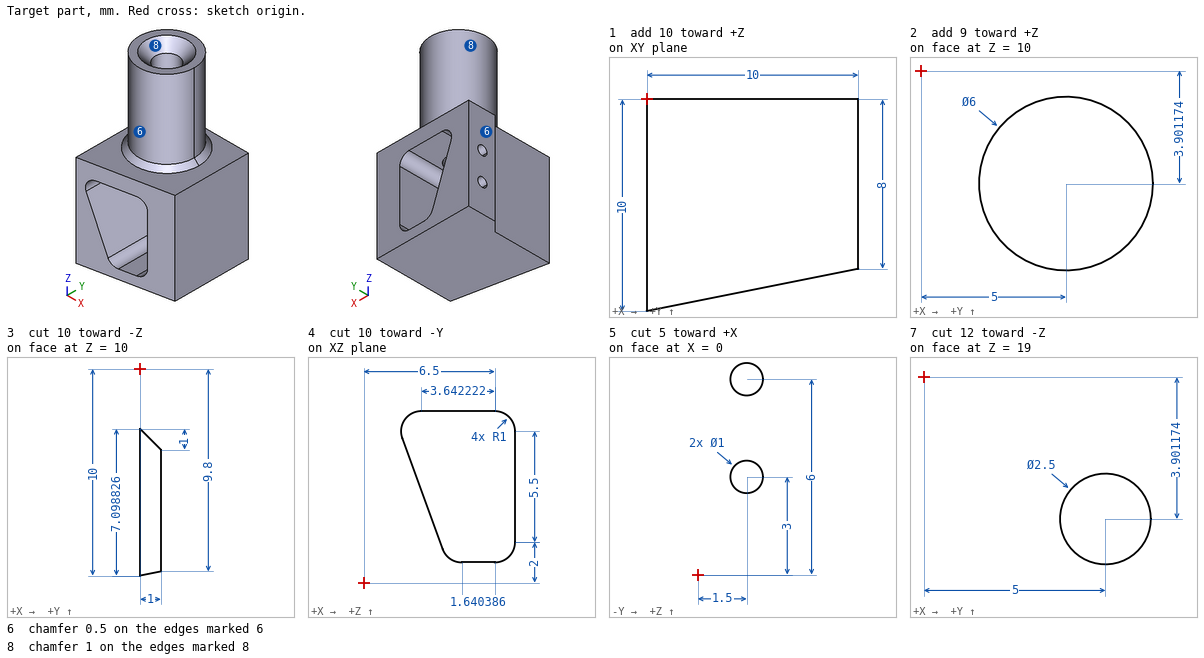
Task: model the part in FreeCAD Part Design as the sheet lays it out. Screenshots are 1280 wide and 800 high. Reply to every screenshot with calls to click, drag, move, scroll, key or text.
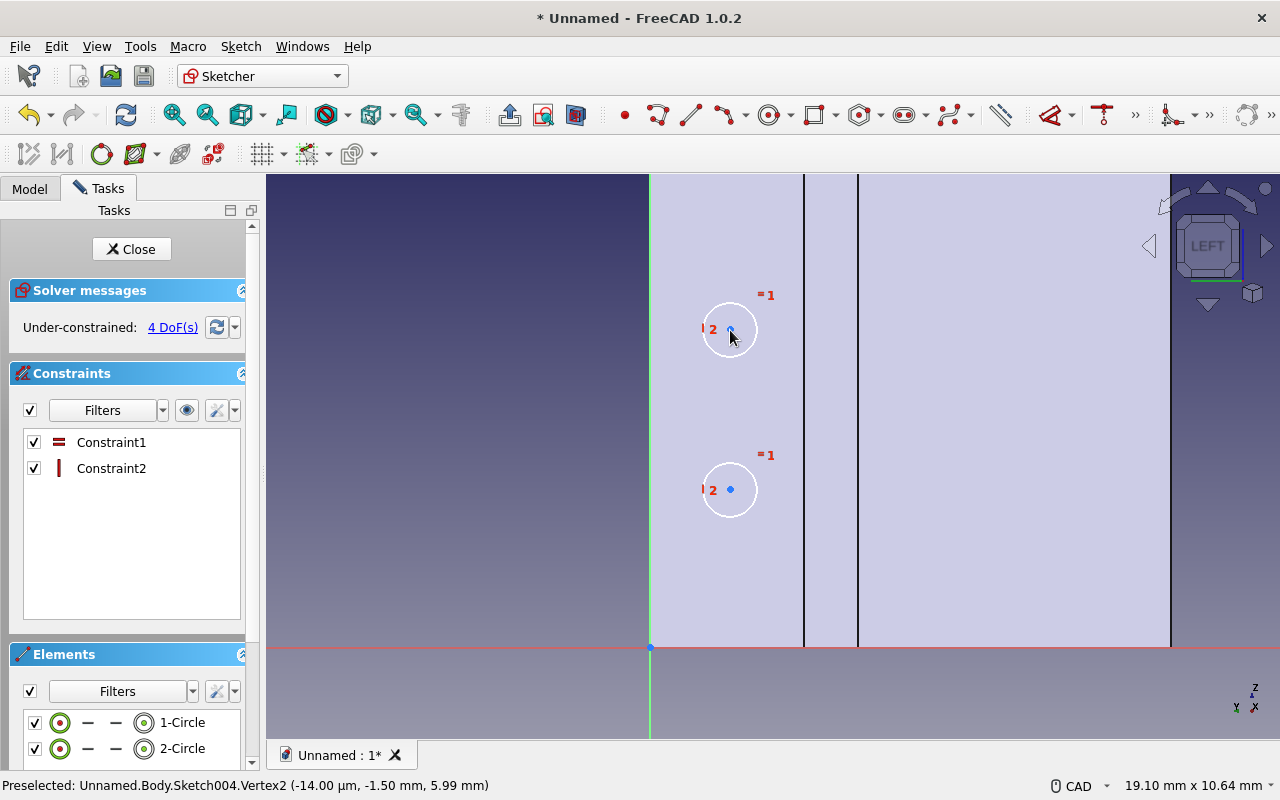
key(d)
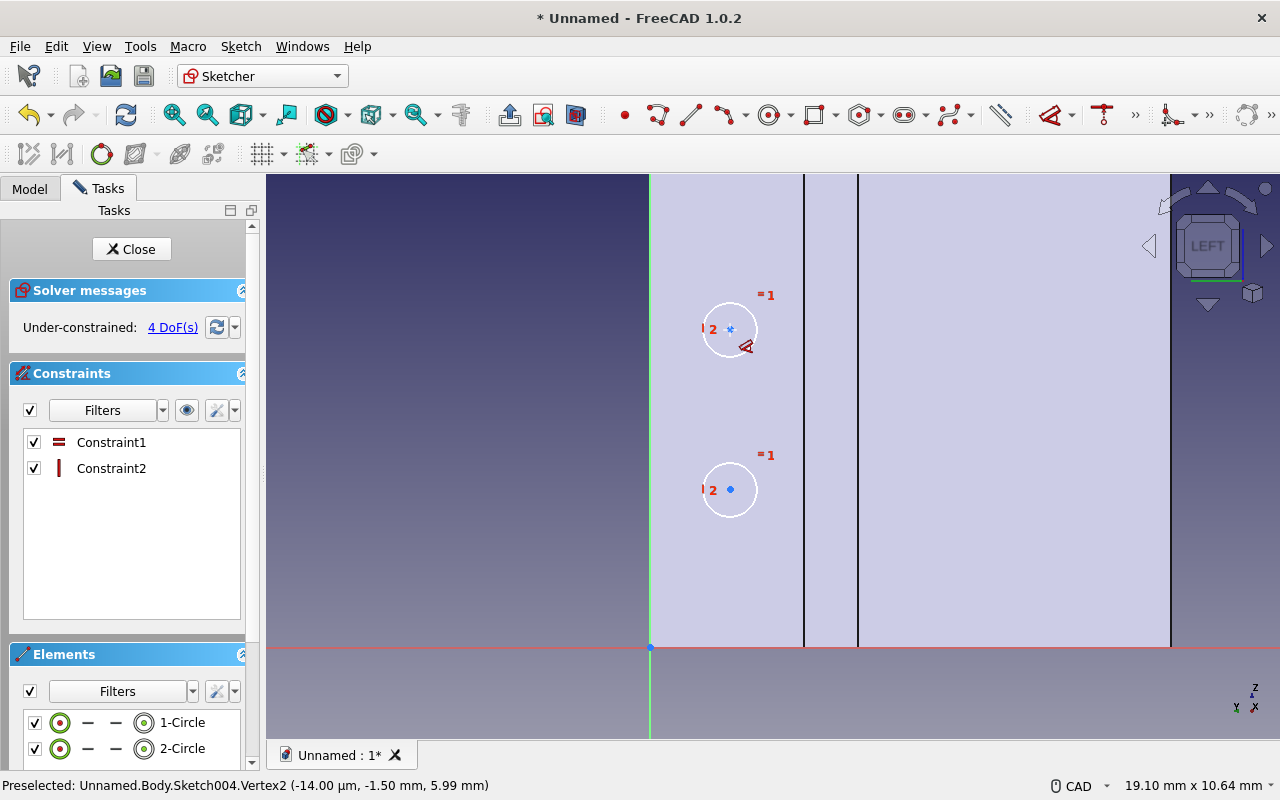
click(749, 471)
click(772, 448)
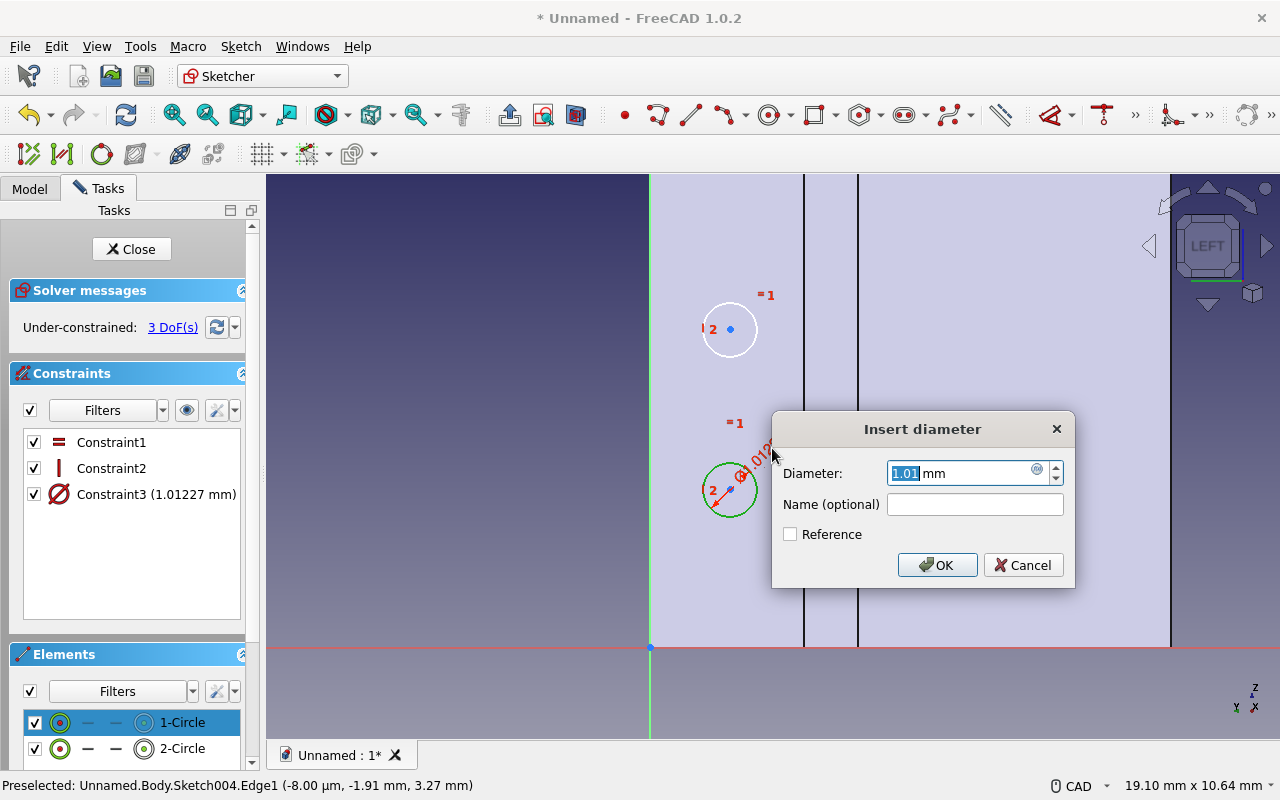
text(1)
key(Return)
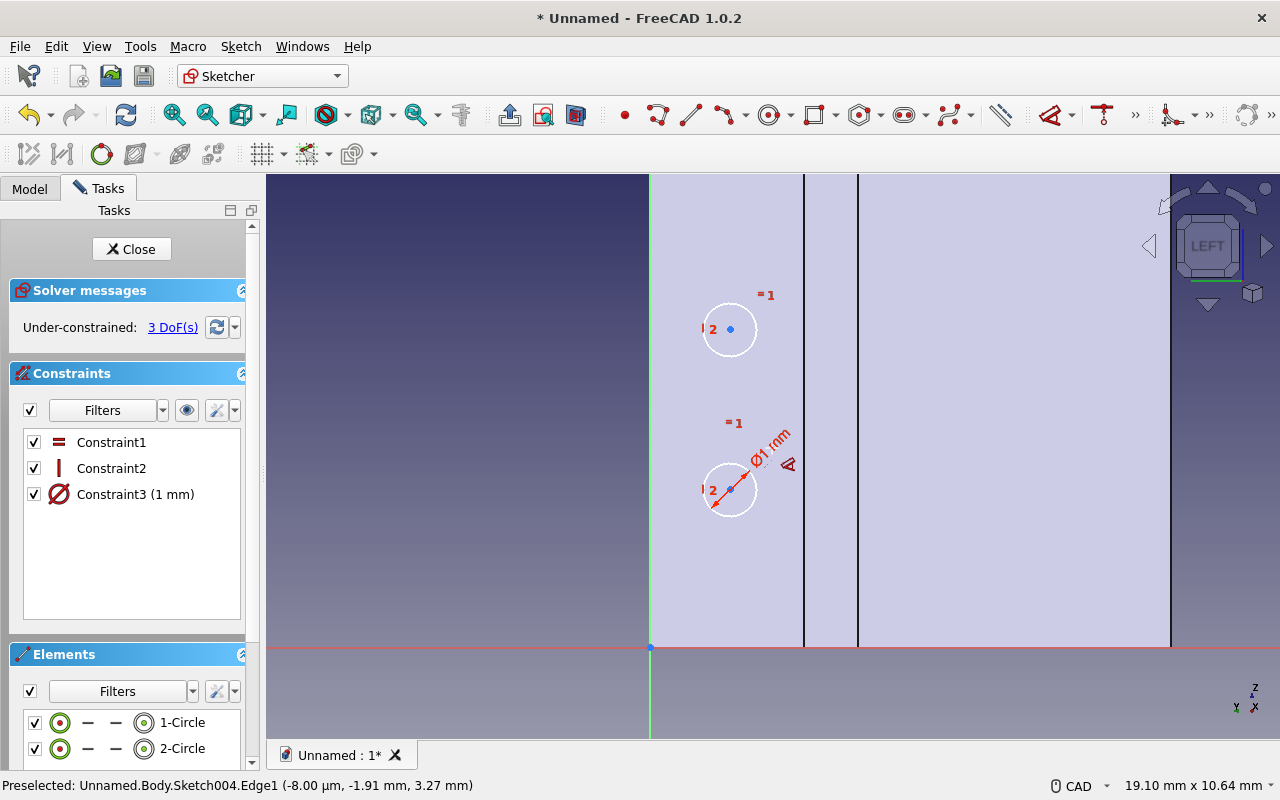
click(730, 490)
click(616, 569)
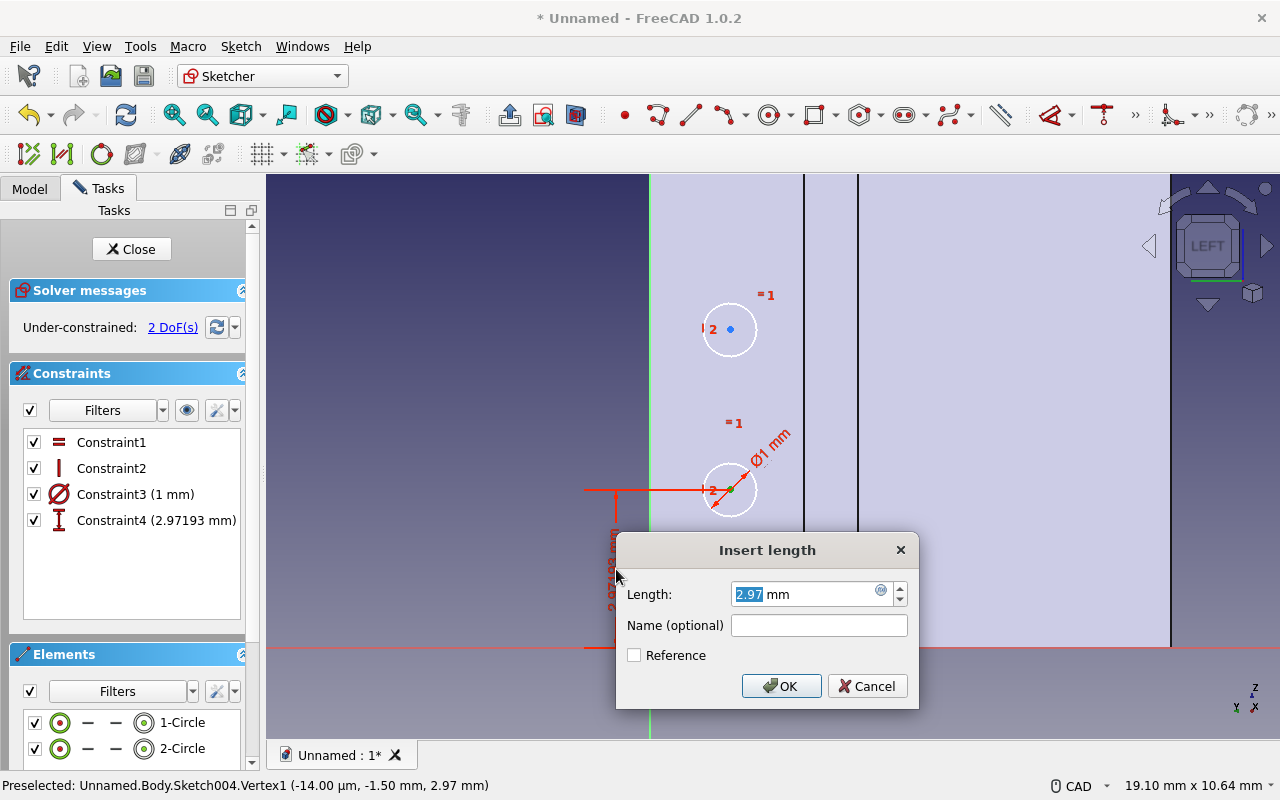
text(3)
key(Return)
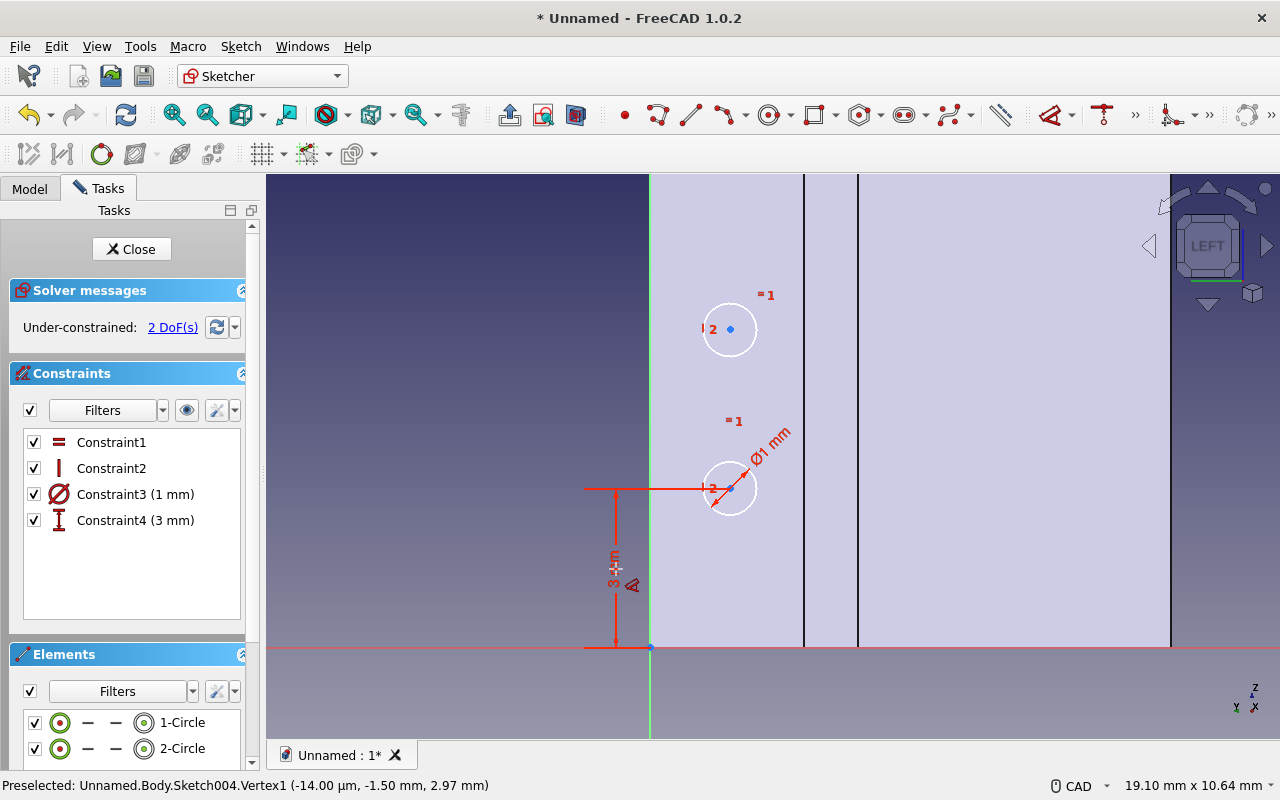
click(730, 330)
click(616, 489)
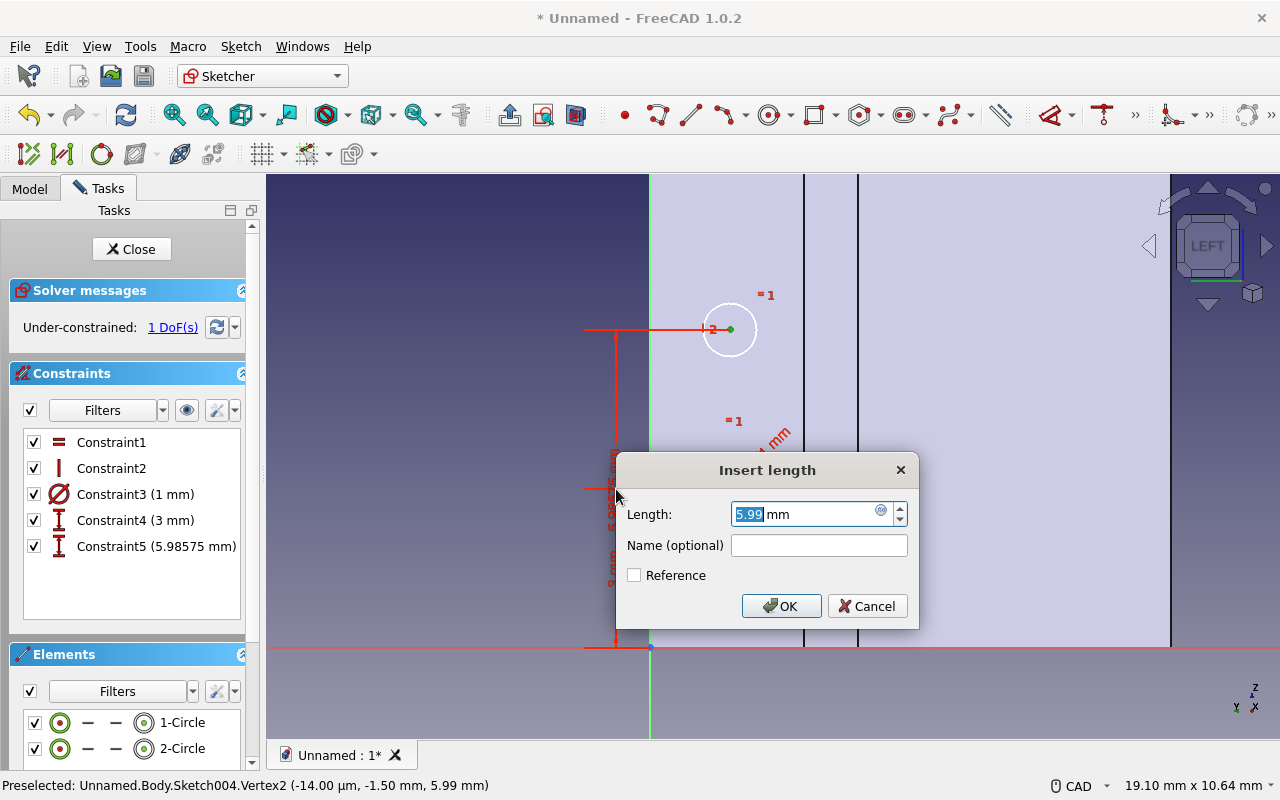
text(6)
key(Return)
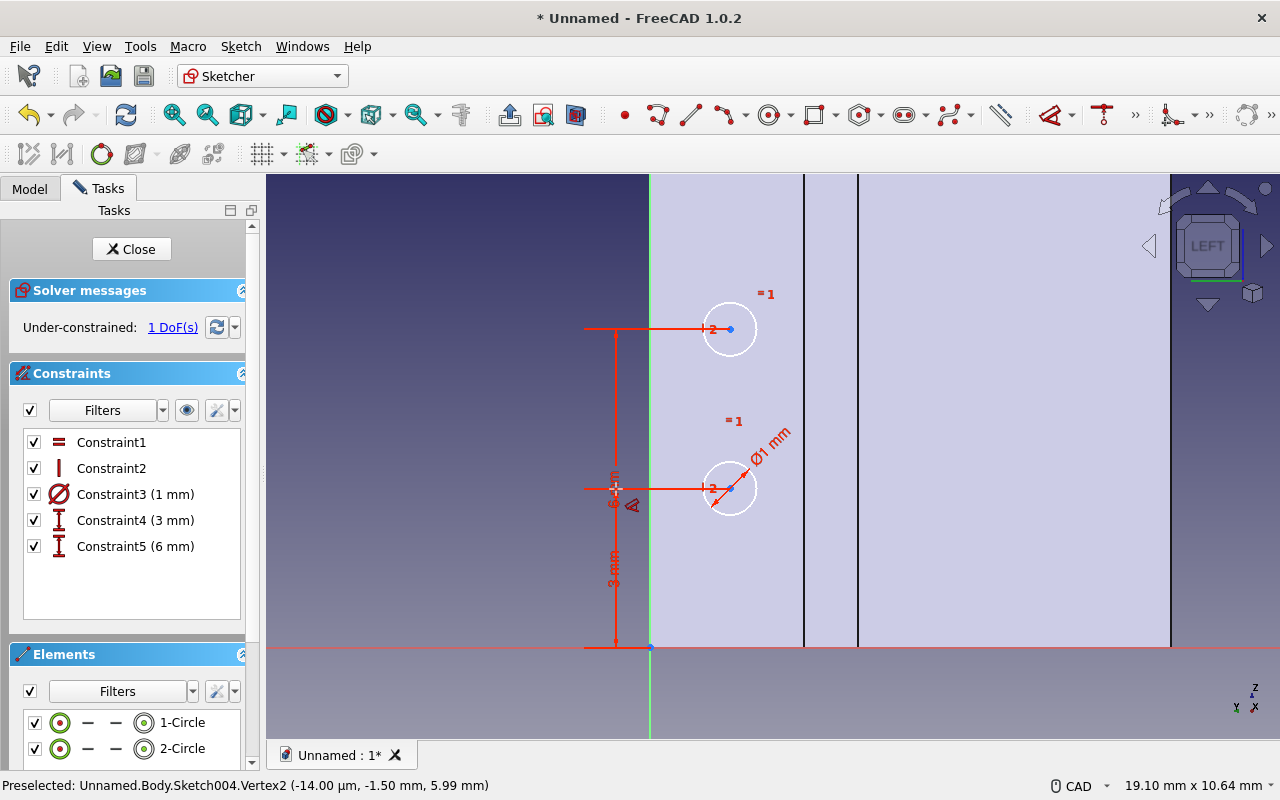
click(730, 489)
click(690, 682)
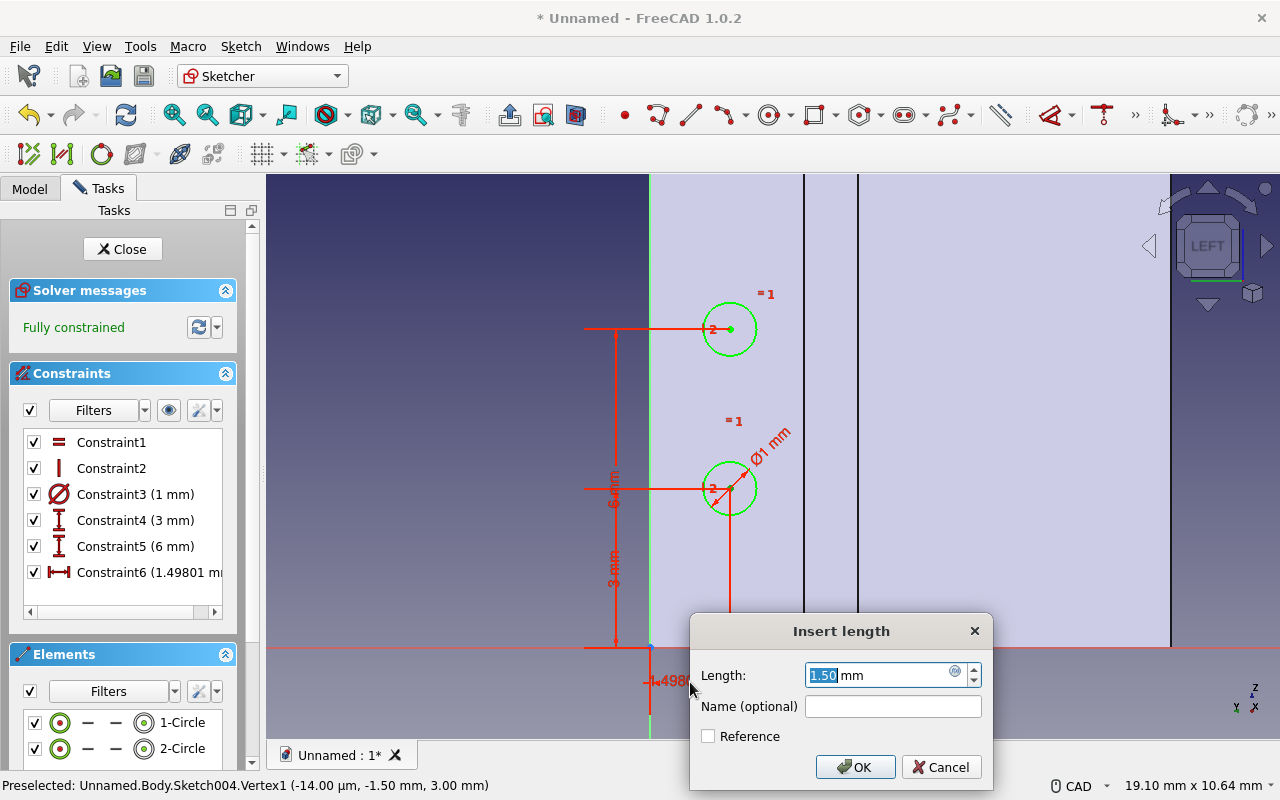
text(1.5)
key(Return)
key(Escape)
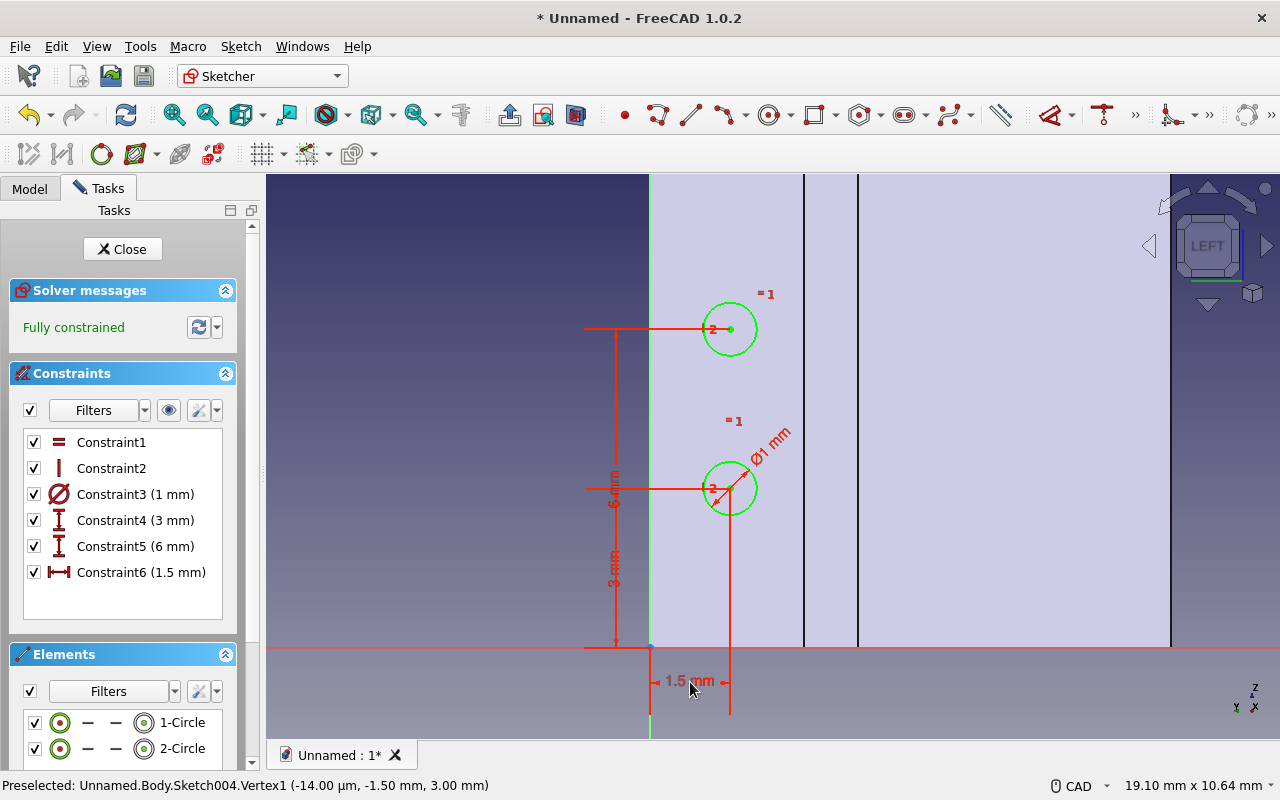
click(123, 249)